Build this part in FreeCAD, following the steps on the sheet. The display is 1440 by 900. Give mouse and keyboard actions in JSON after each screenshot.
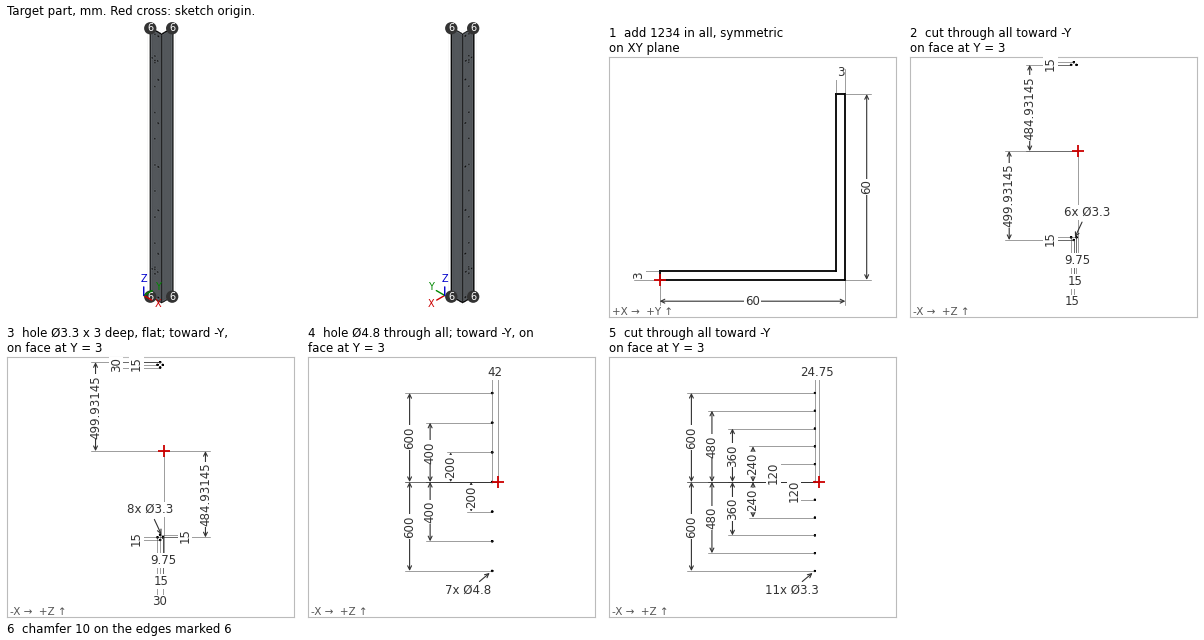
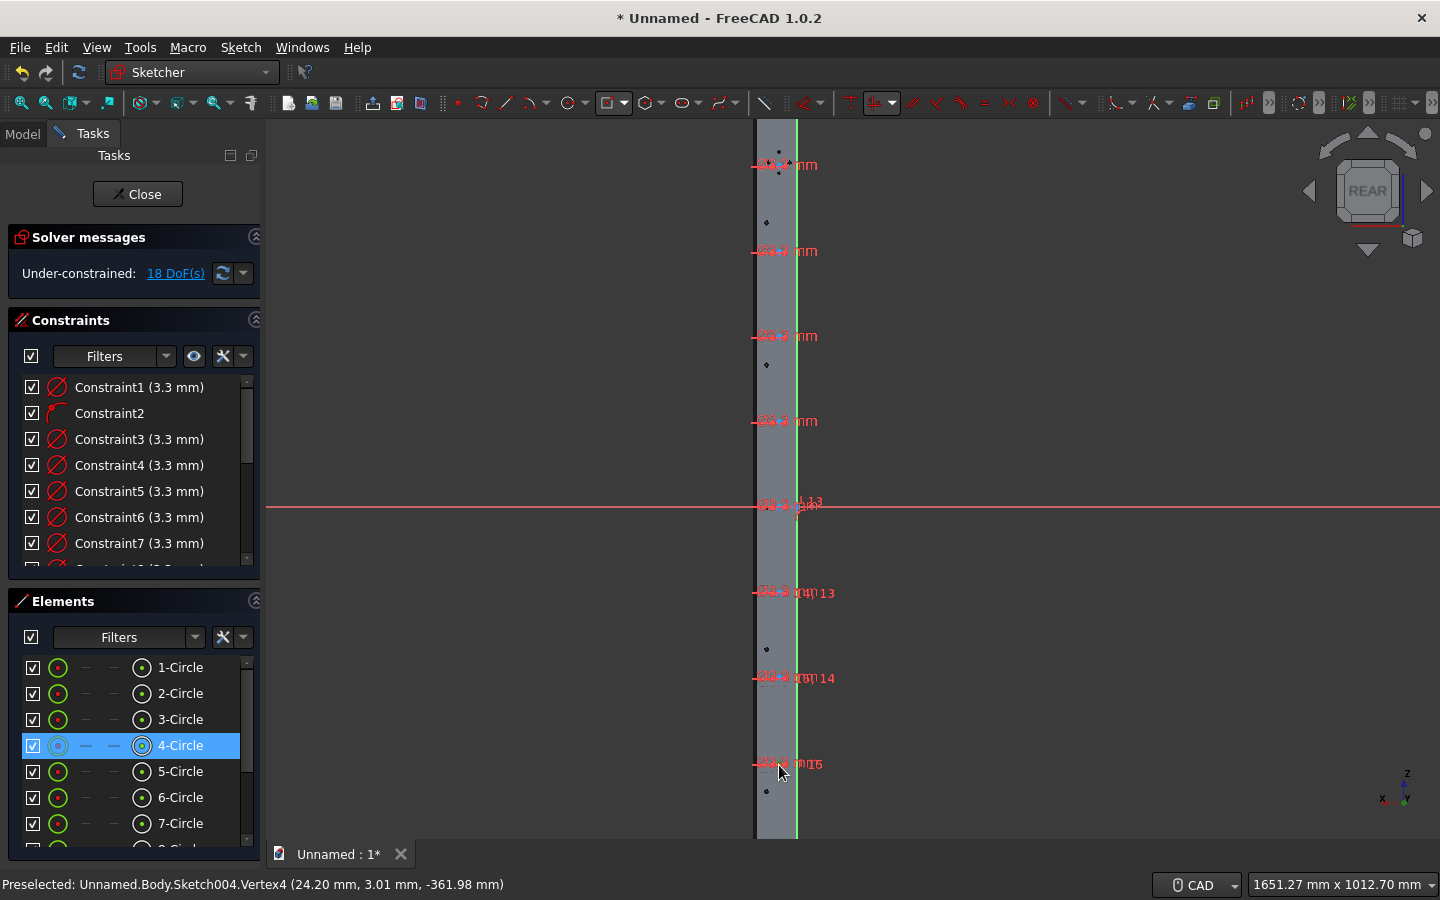
{"action": "scroll", "coordinate": [781, 445], "scroll_direction": "down", "scroll_amount": 3}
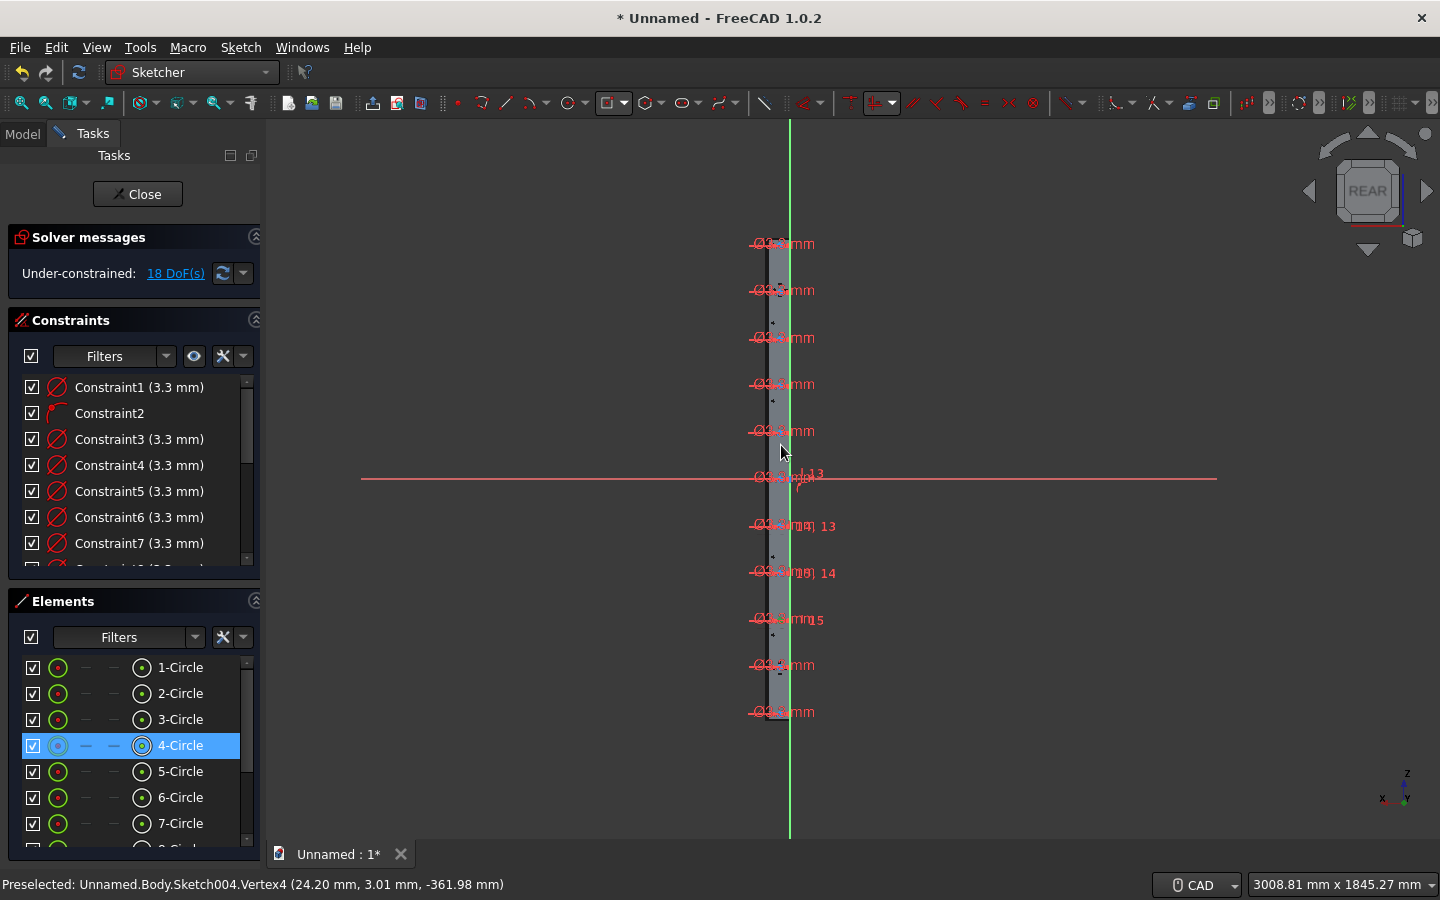
{"action": "left_click", "coordinate": [780, 667]}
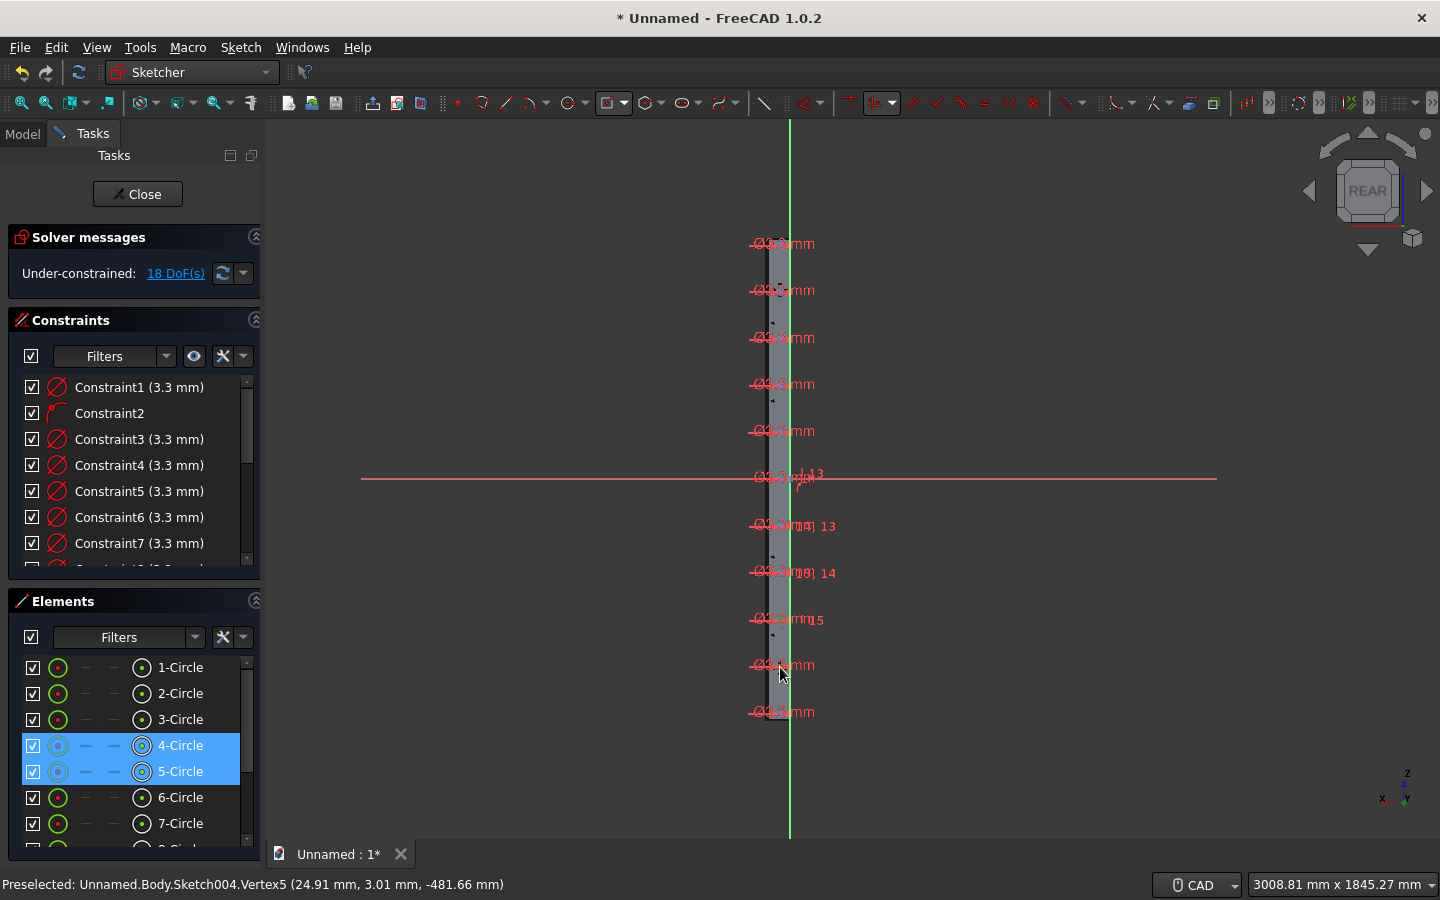
{"action": "key", "text": "v"}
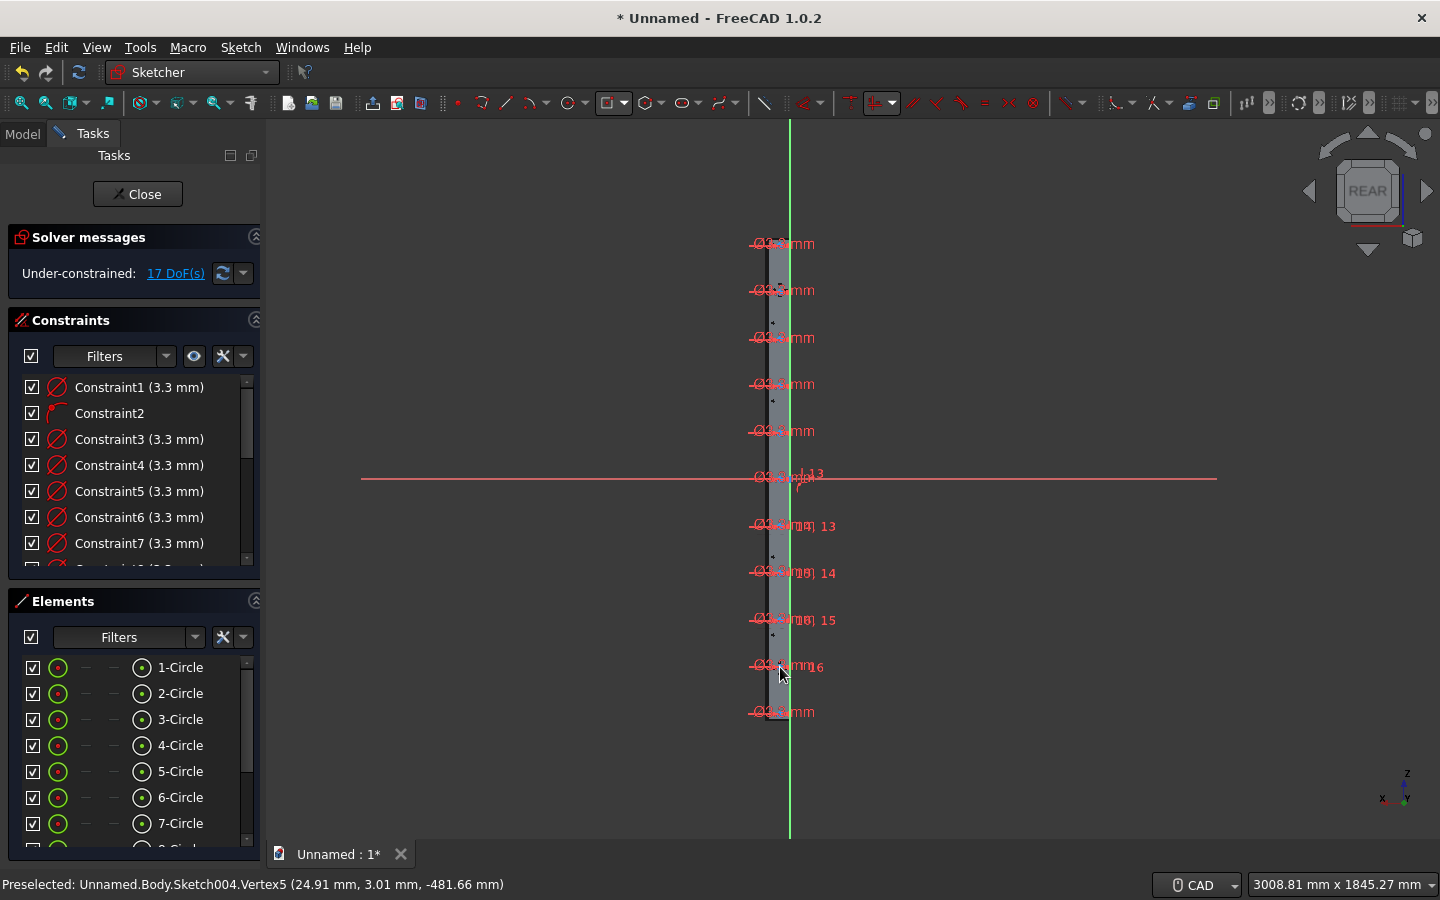
{"action": "left_click", "coordinate": [780, 667]}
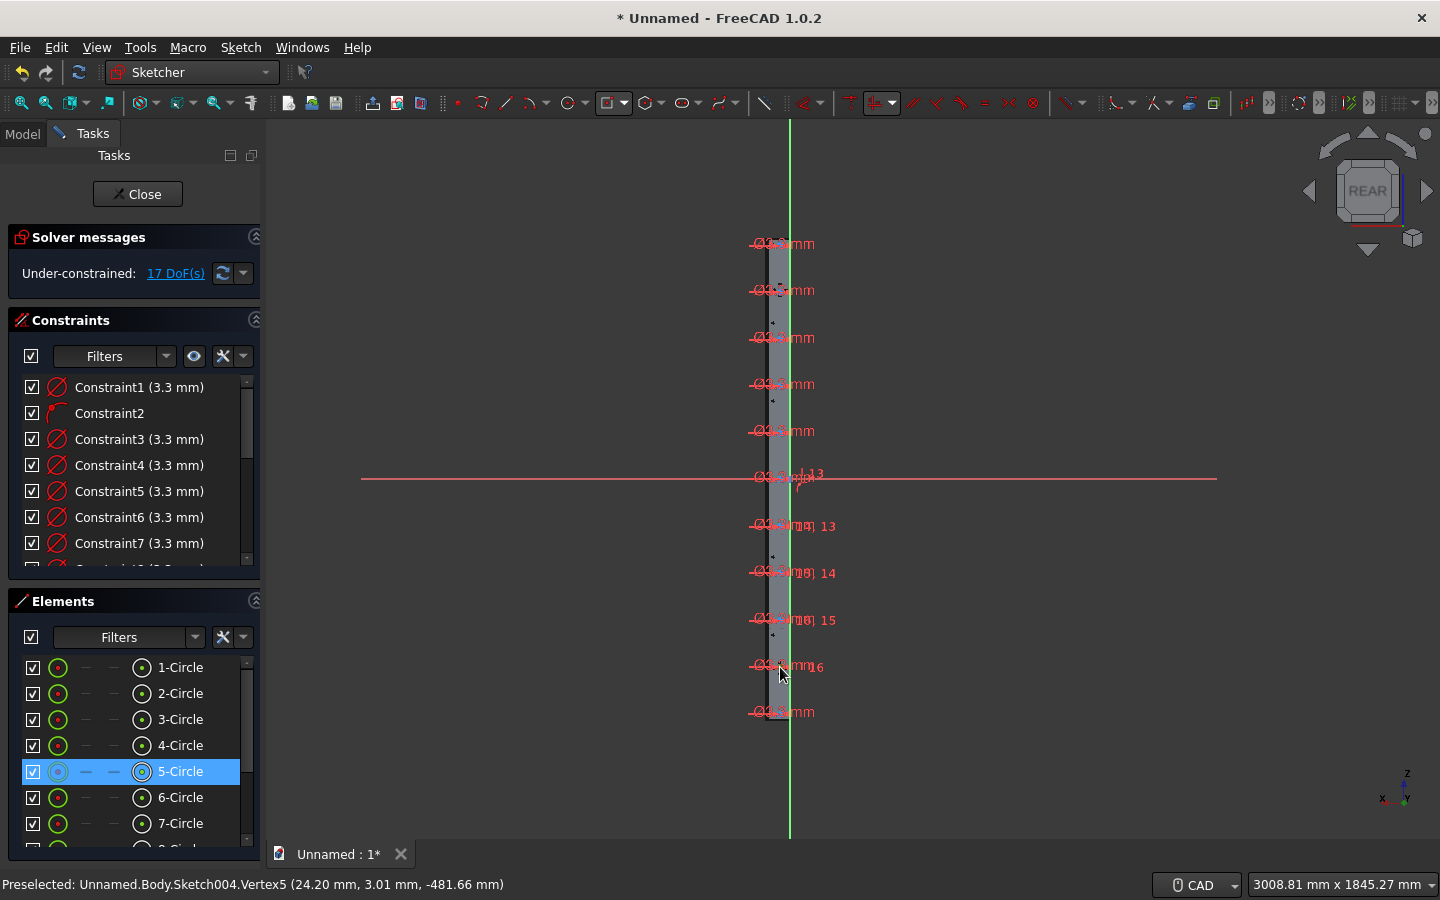
{"action": "left_click", "coordinate": [780, 714]}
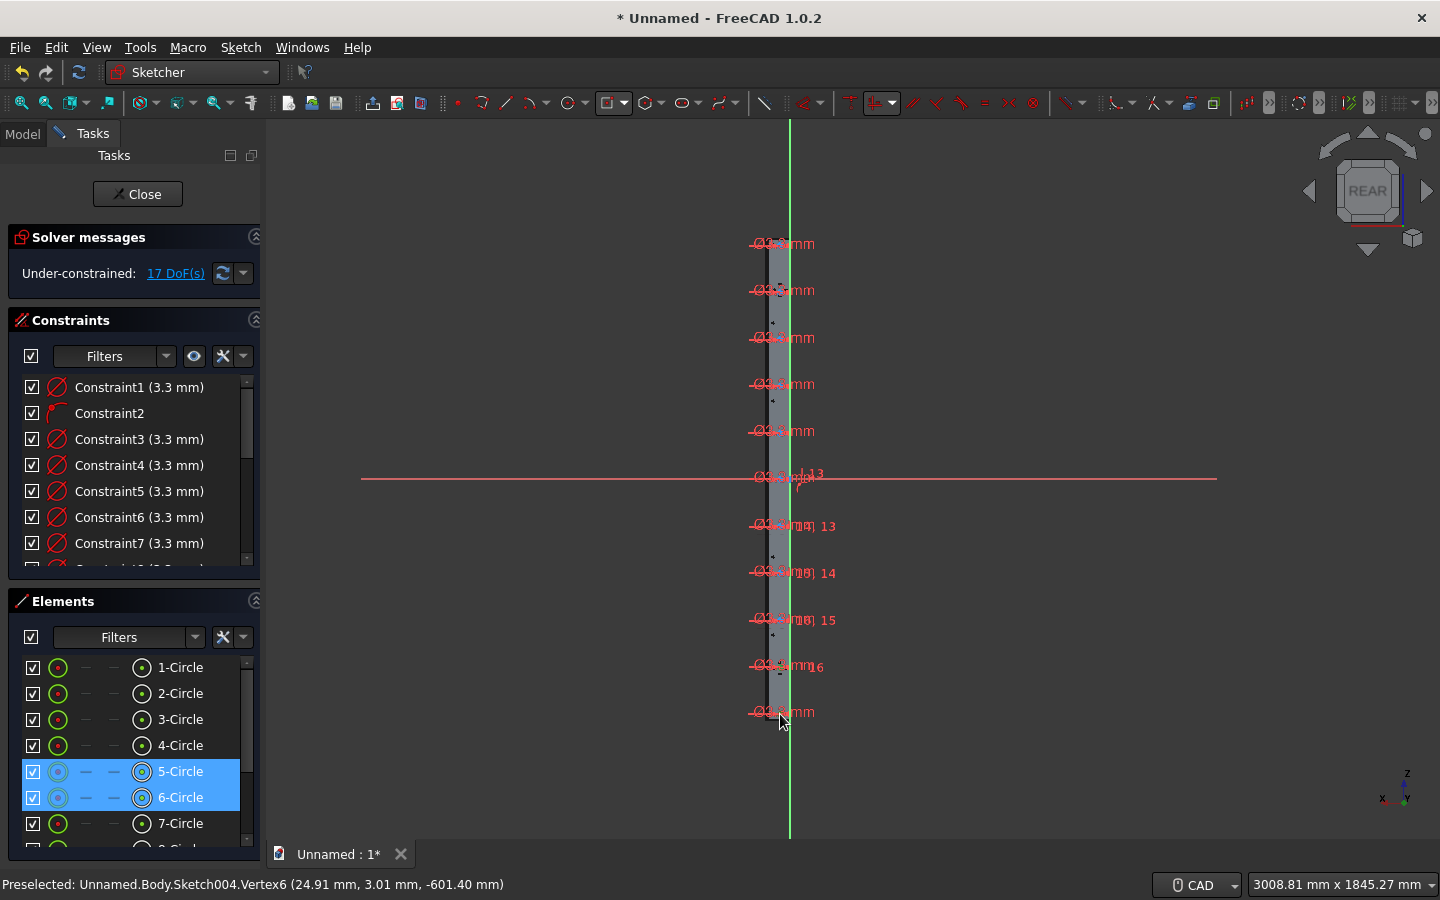
{"action": "key", "text": "v"}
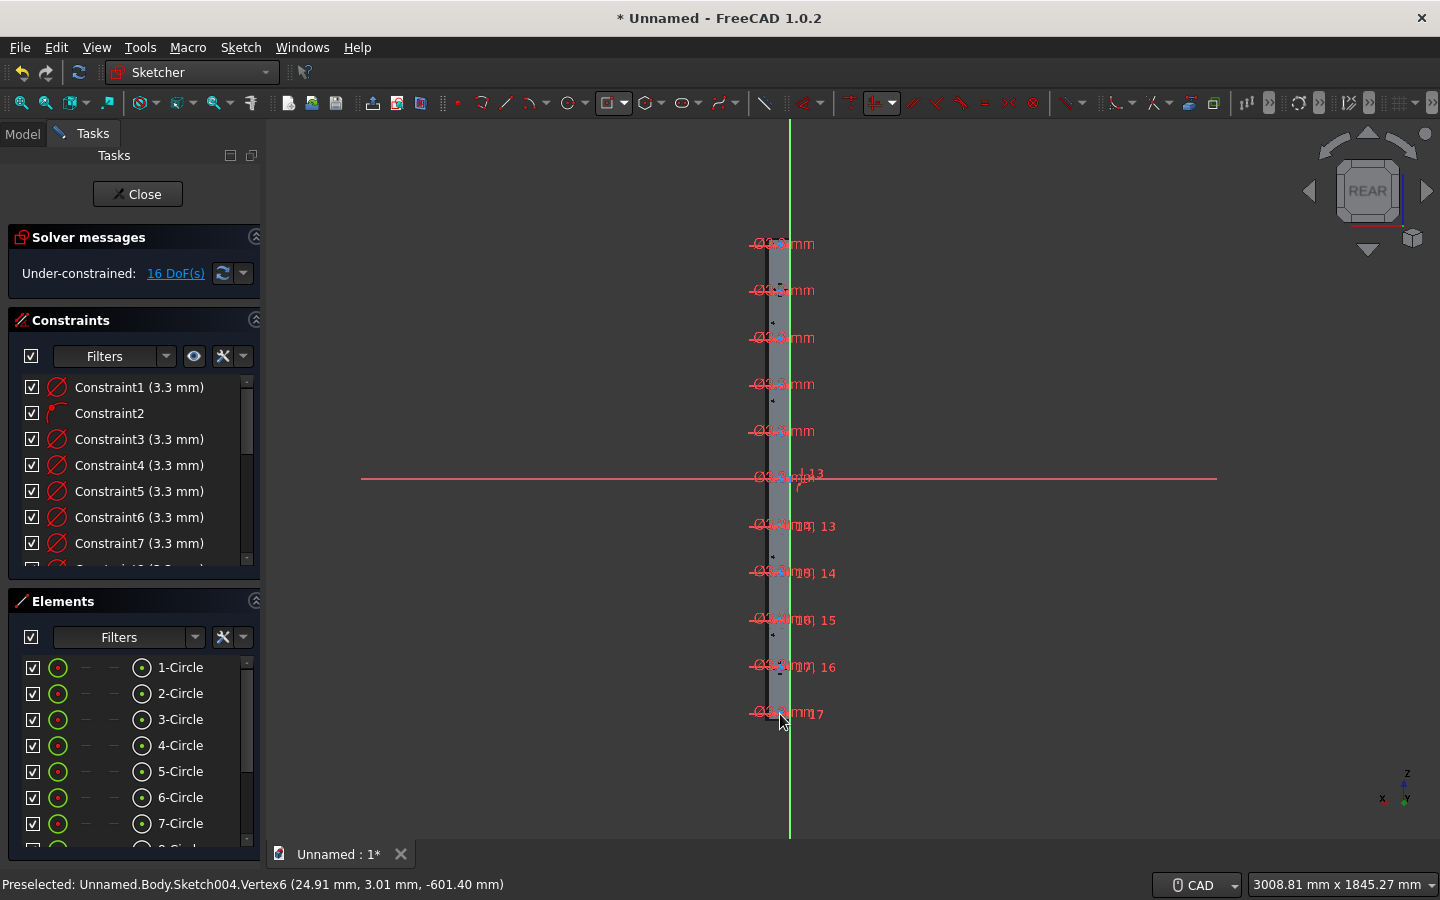
{"action": "scroll", "coordinate": [780, 479], "scroll_direction": "up", "scroll_amount": 2}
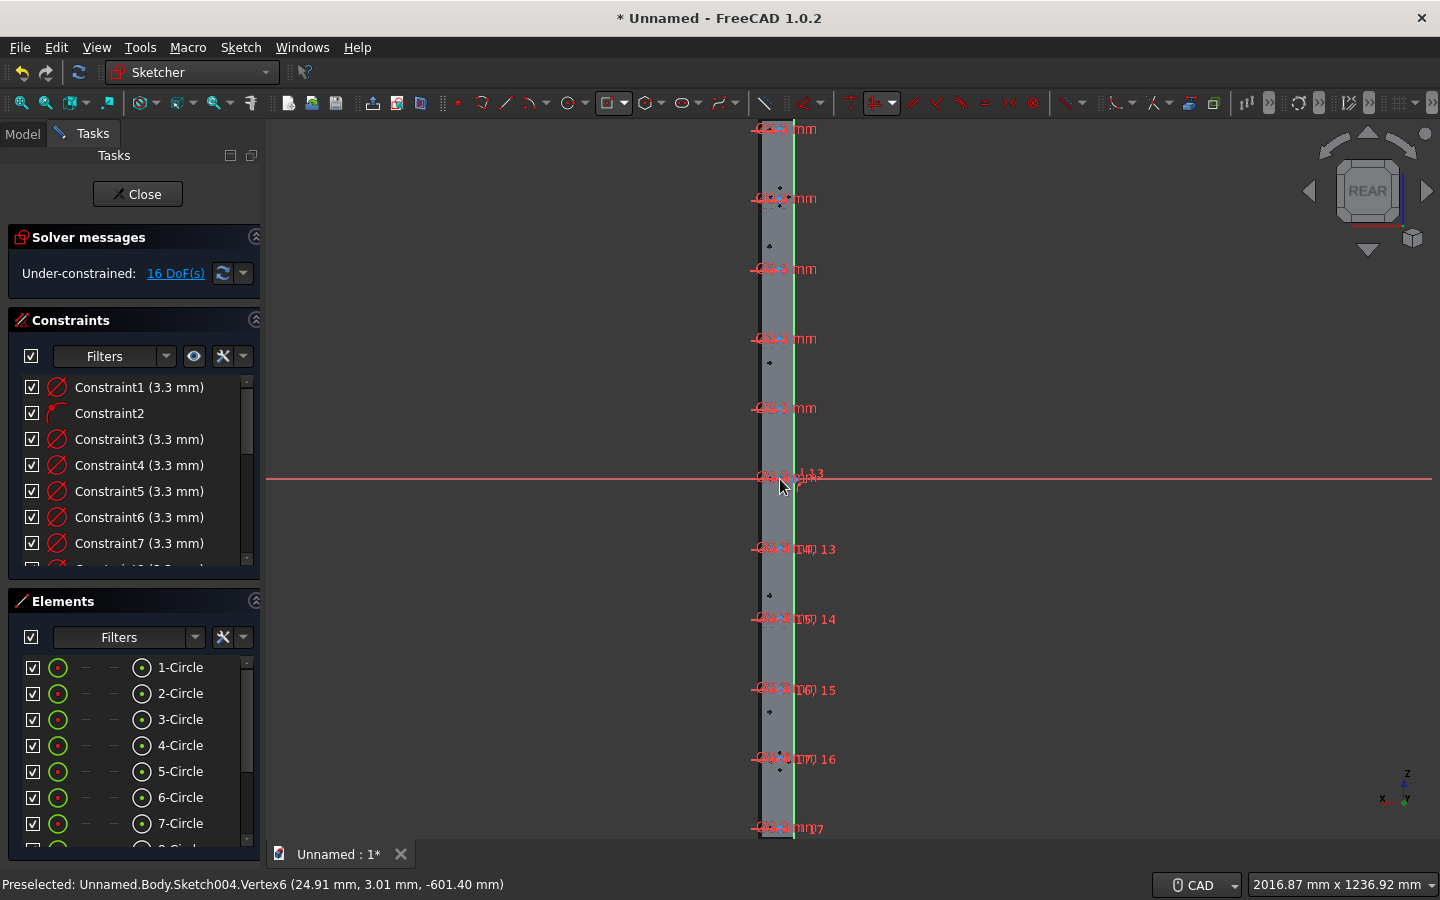
{"action": "left_click", "coordinate": [780, 479]}